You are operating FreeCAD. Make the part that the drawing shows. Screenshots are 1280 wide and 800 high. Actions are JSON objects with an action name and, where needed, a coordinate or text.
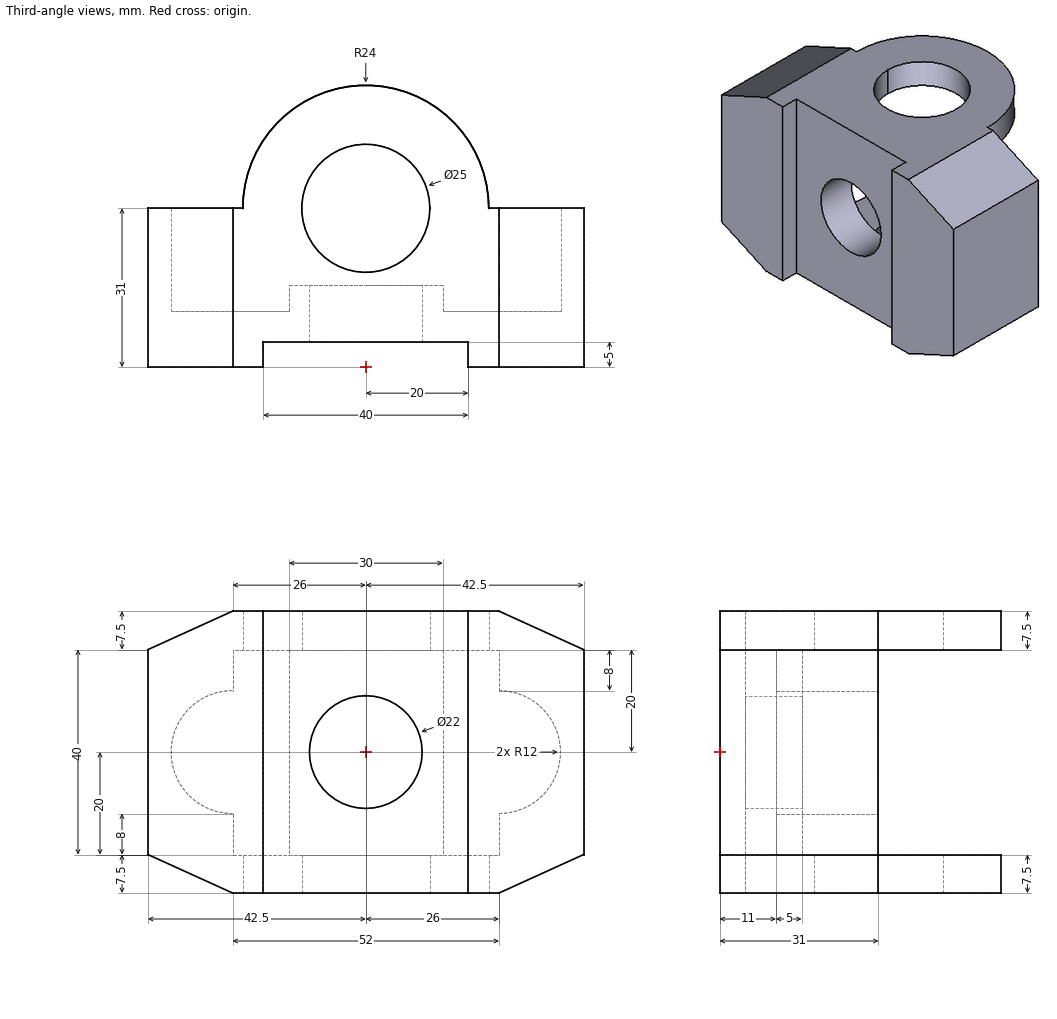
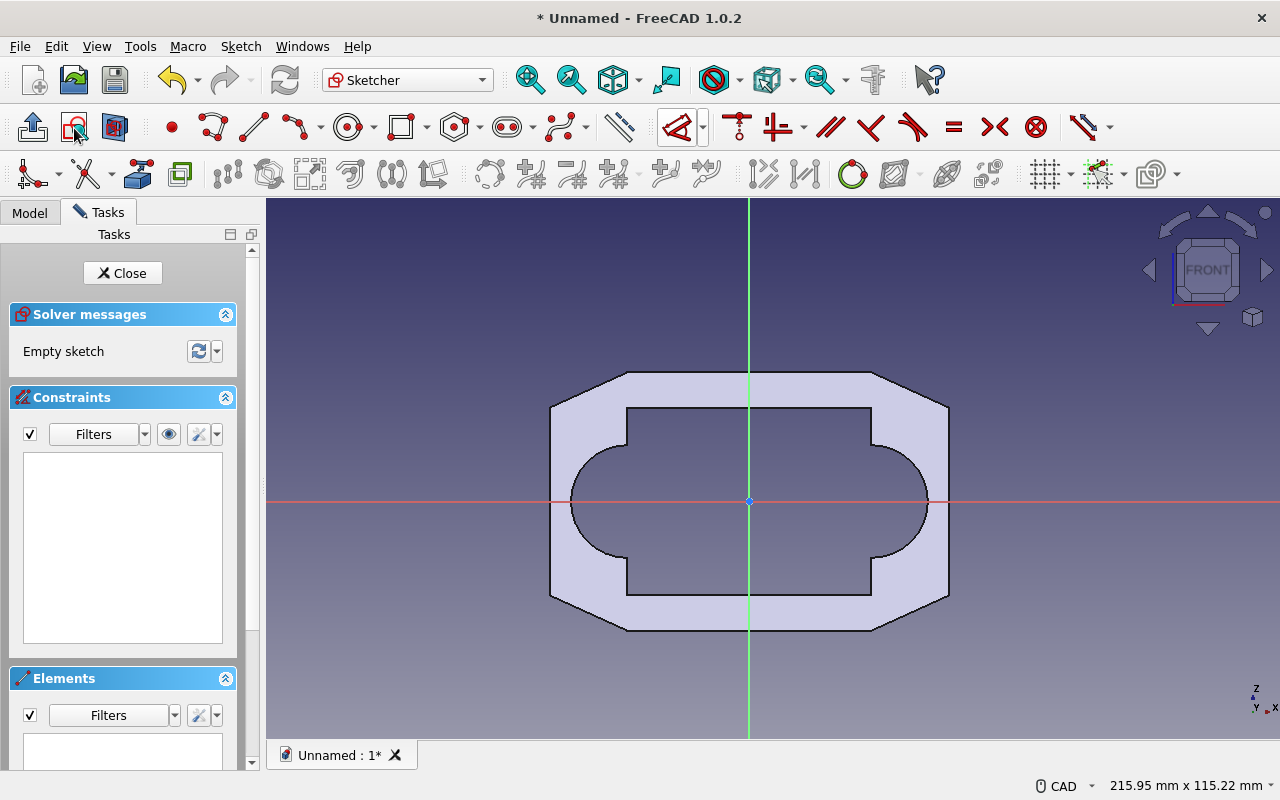
{"action": "left_click", "coordinate": [871, 631]}
{"action": "left_click", "coordinate": [627, 631]}
{"action": "left_click", "coordinate": [550, 595]}
{"action": "left_click", "coordinate": [550, 408]}
{"action": "left_click", "coordinate": [627, 372]}
{"action": "left_click", "coordinate": [871, 372]}
{"action": "left_click", "coordinate": [949, 408]}
{"action": "left_click", "coordinate": [949, 595]}
{"action": "left_click", "coordinate": [871, 632]}
{"action": "key", "text": "Escape"}
{"action": "key", "text": "Escape"}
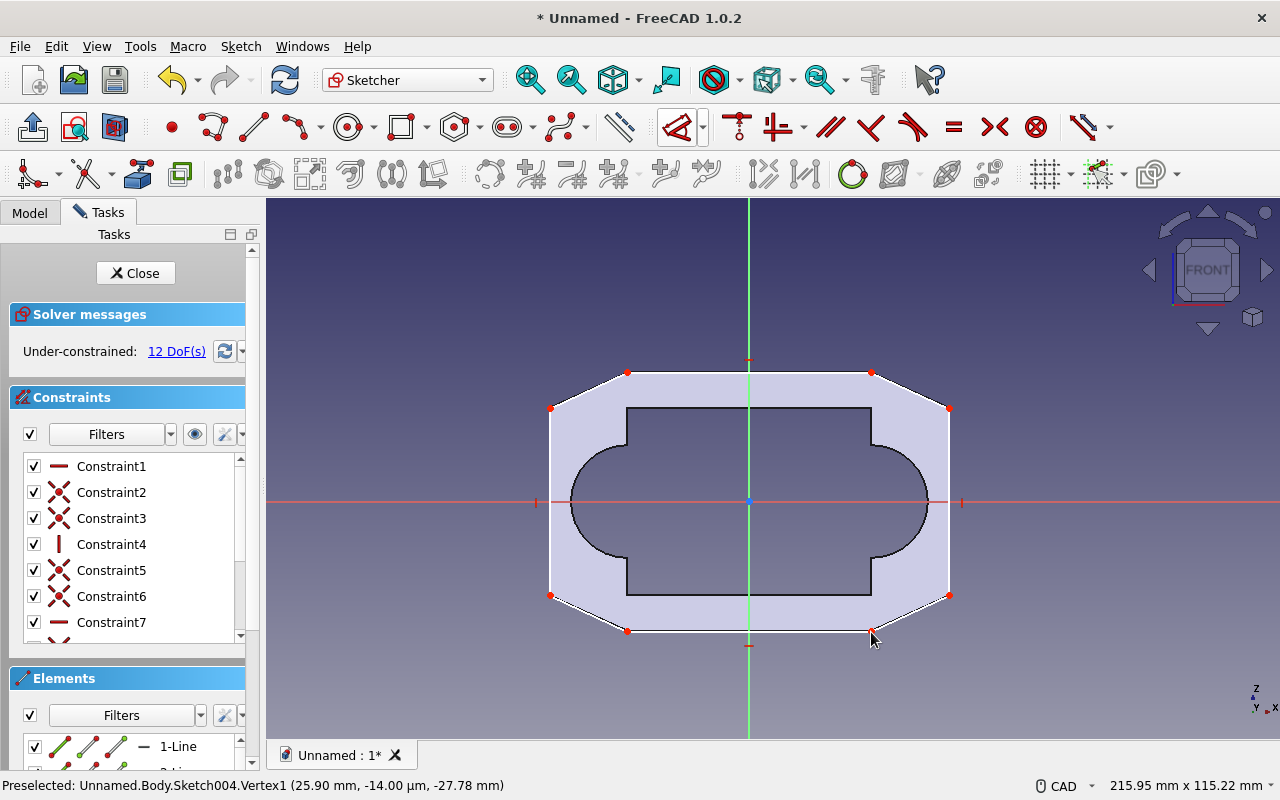
{"action": "left_click", "coordinate": [798, 632]}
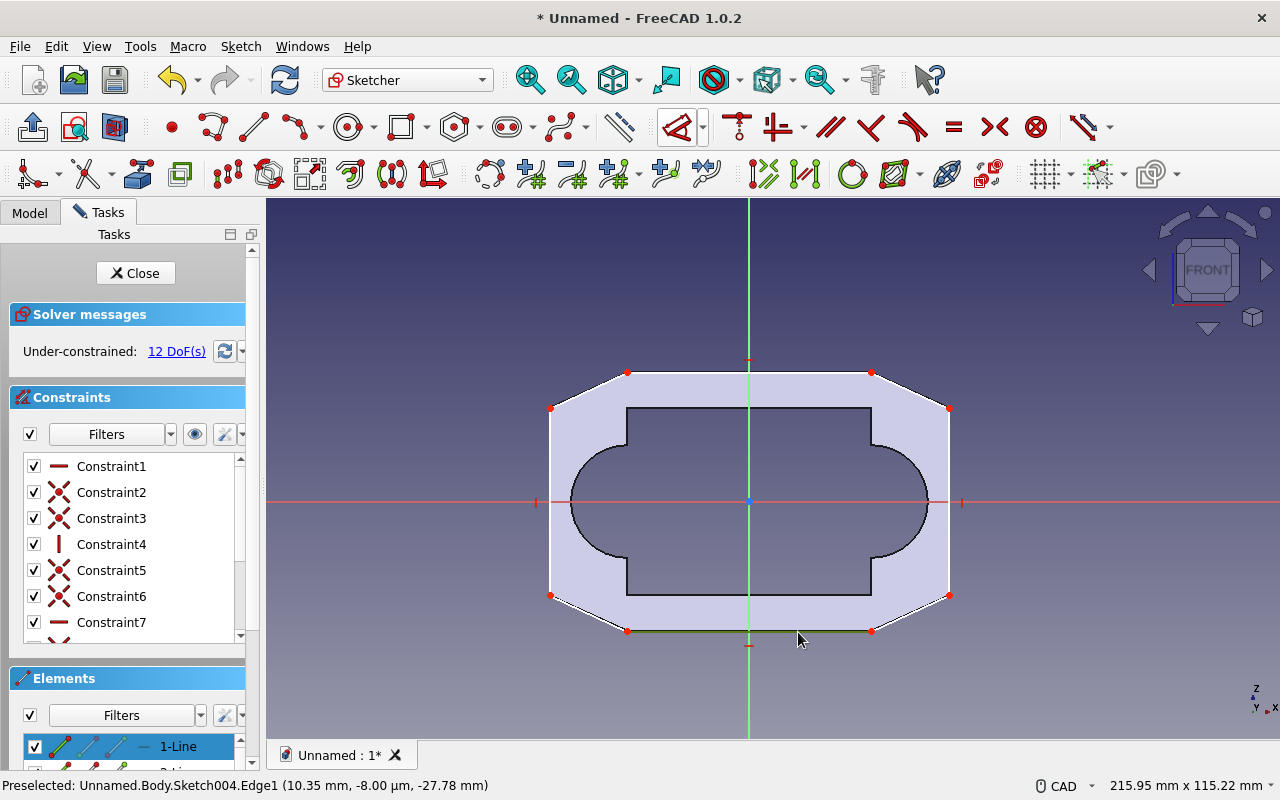
{"action": "key", "text": "l"}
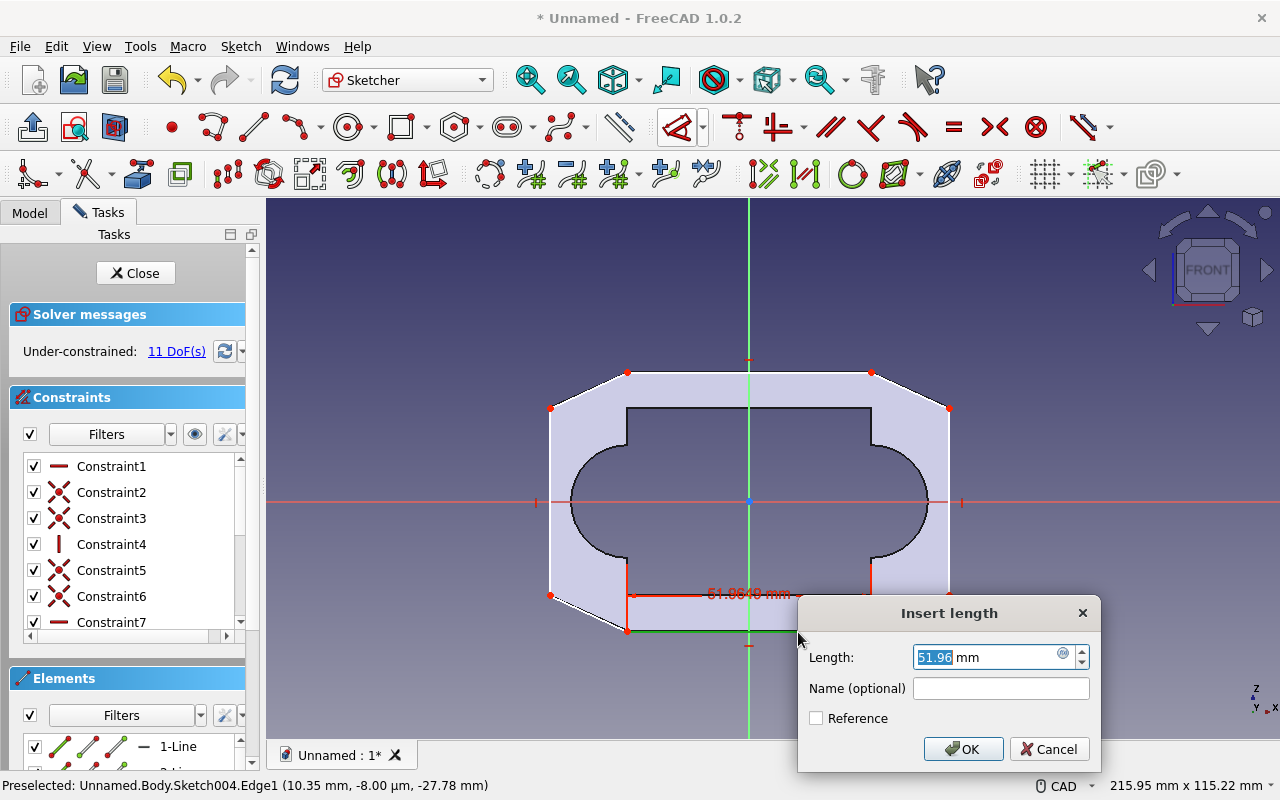
{"action": "type", "text": "52"}
{"action": "key", "text": "Return"}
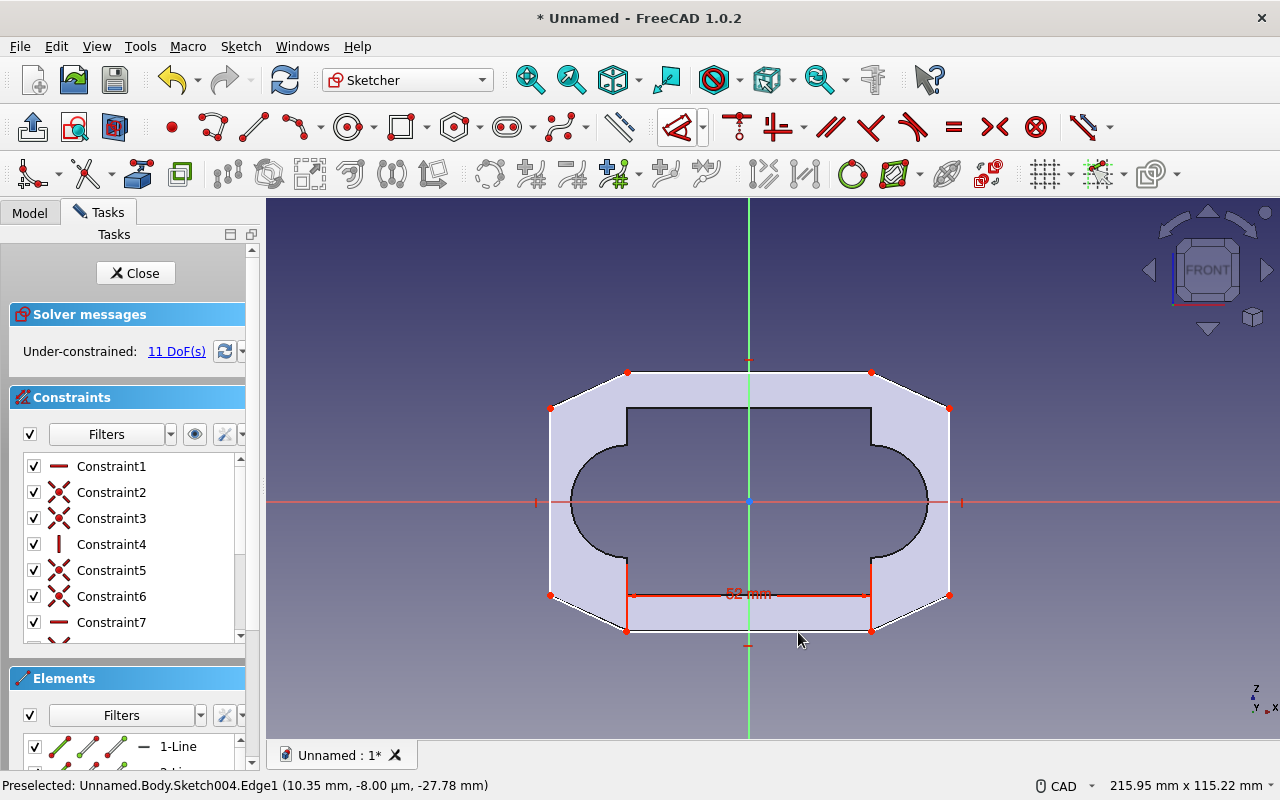
{"action": "left_click", "coordinate": [550, 540]}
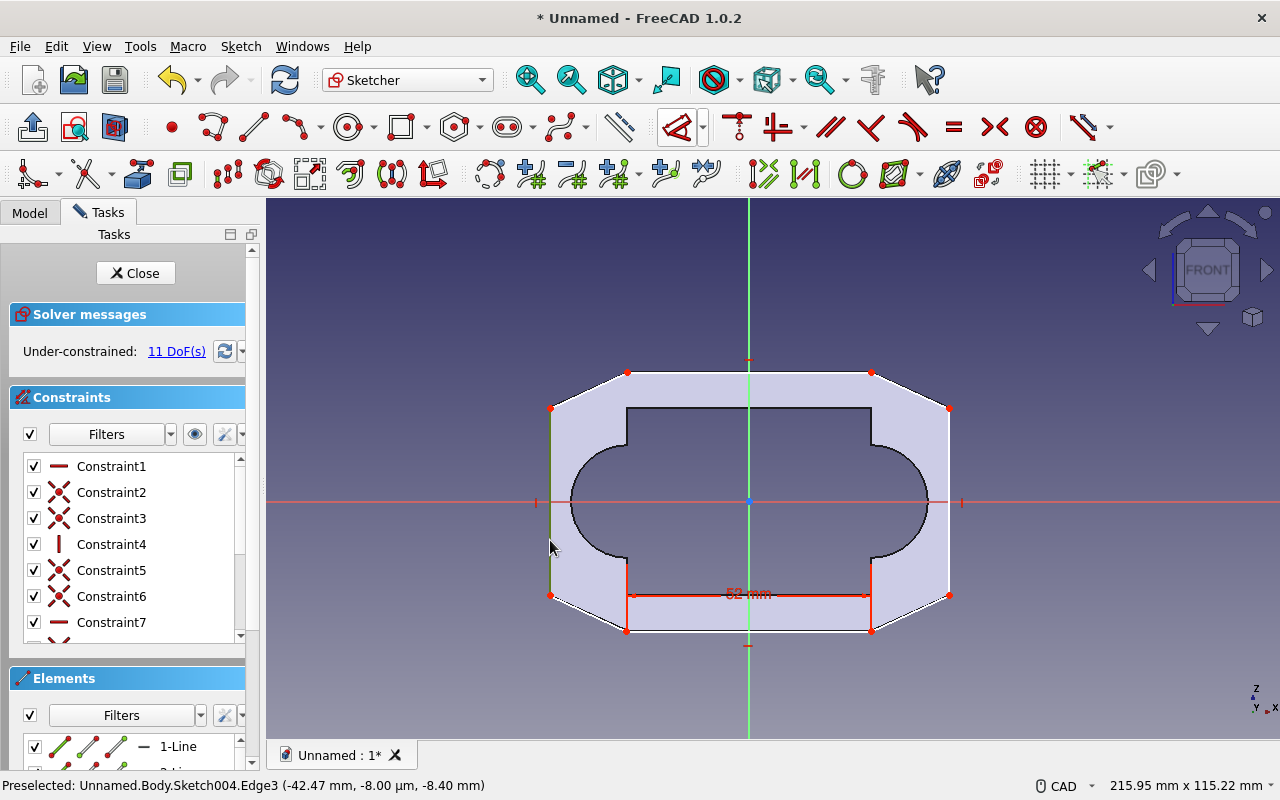
{"action": "key", "text": "i"}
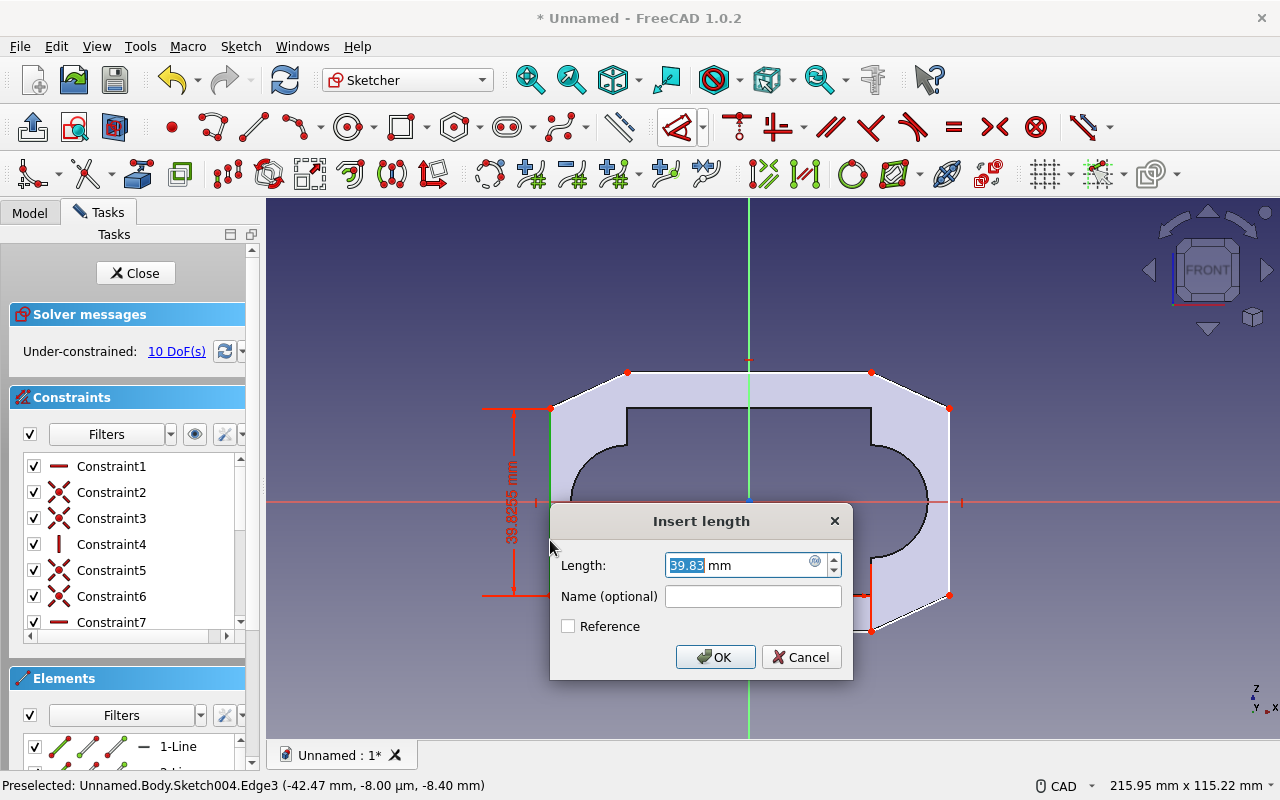
{"action": "type", "text": "40"}
{"action": "key", "text": "Return"}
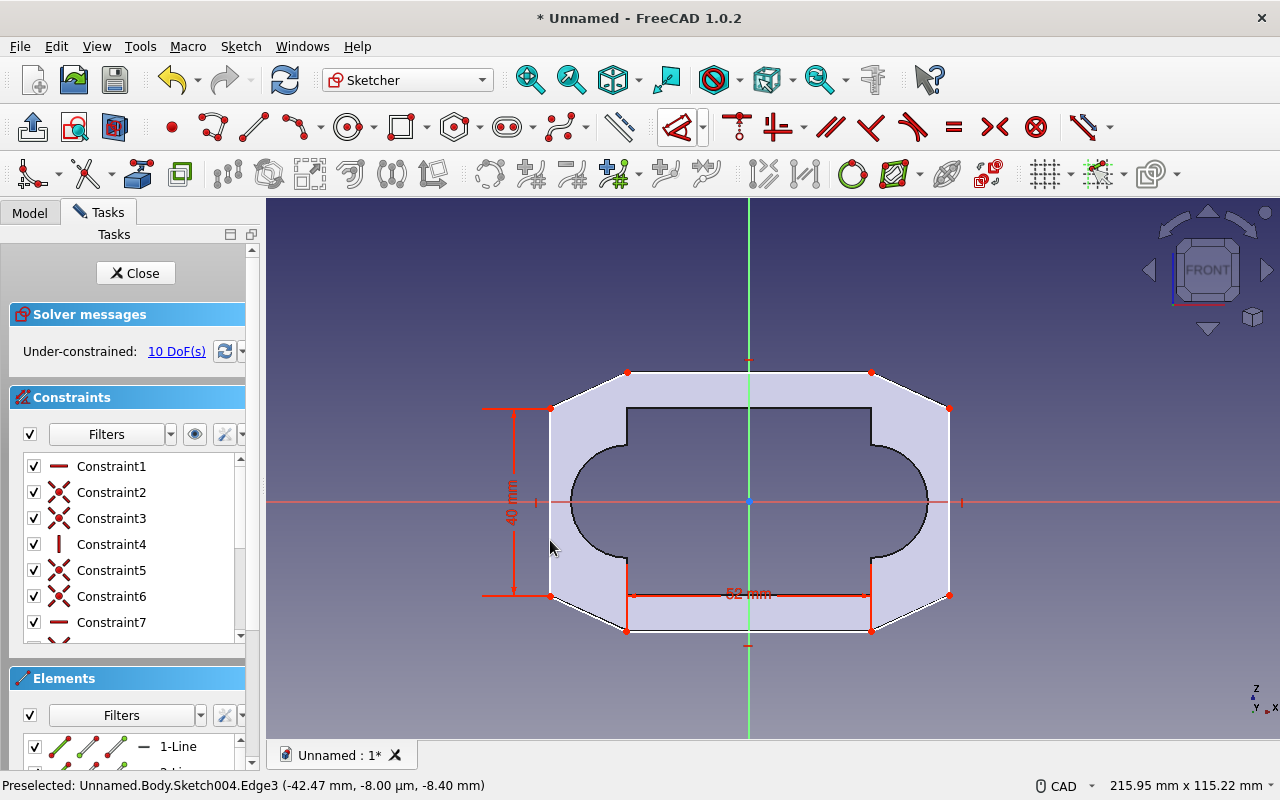
{"action": "left_click", "coordinate": [700, 373]}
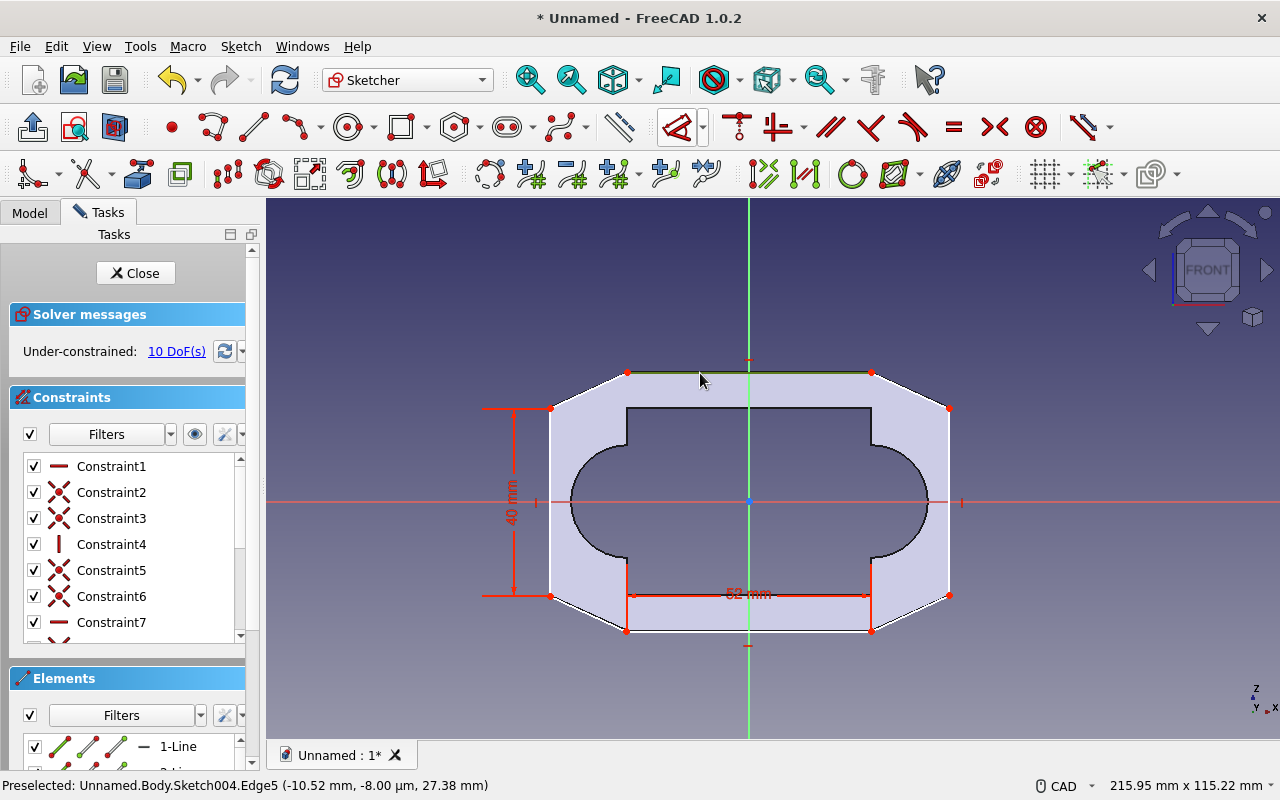
{"action": "key", "text": "l"}